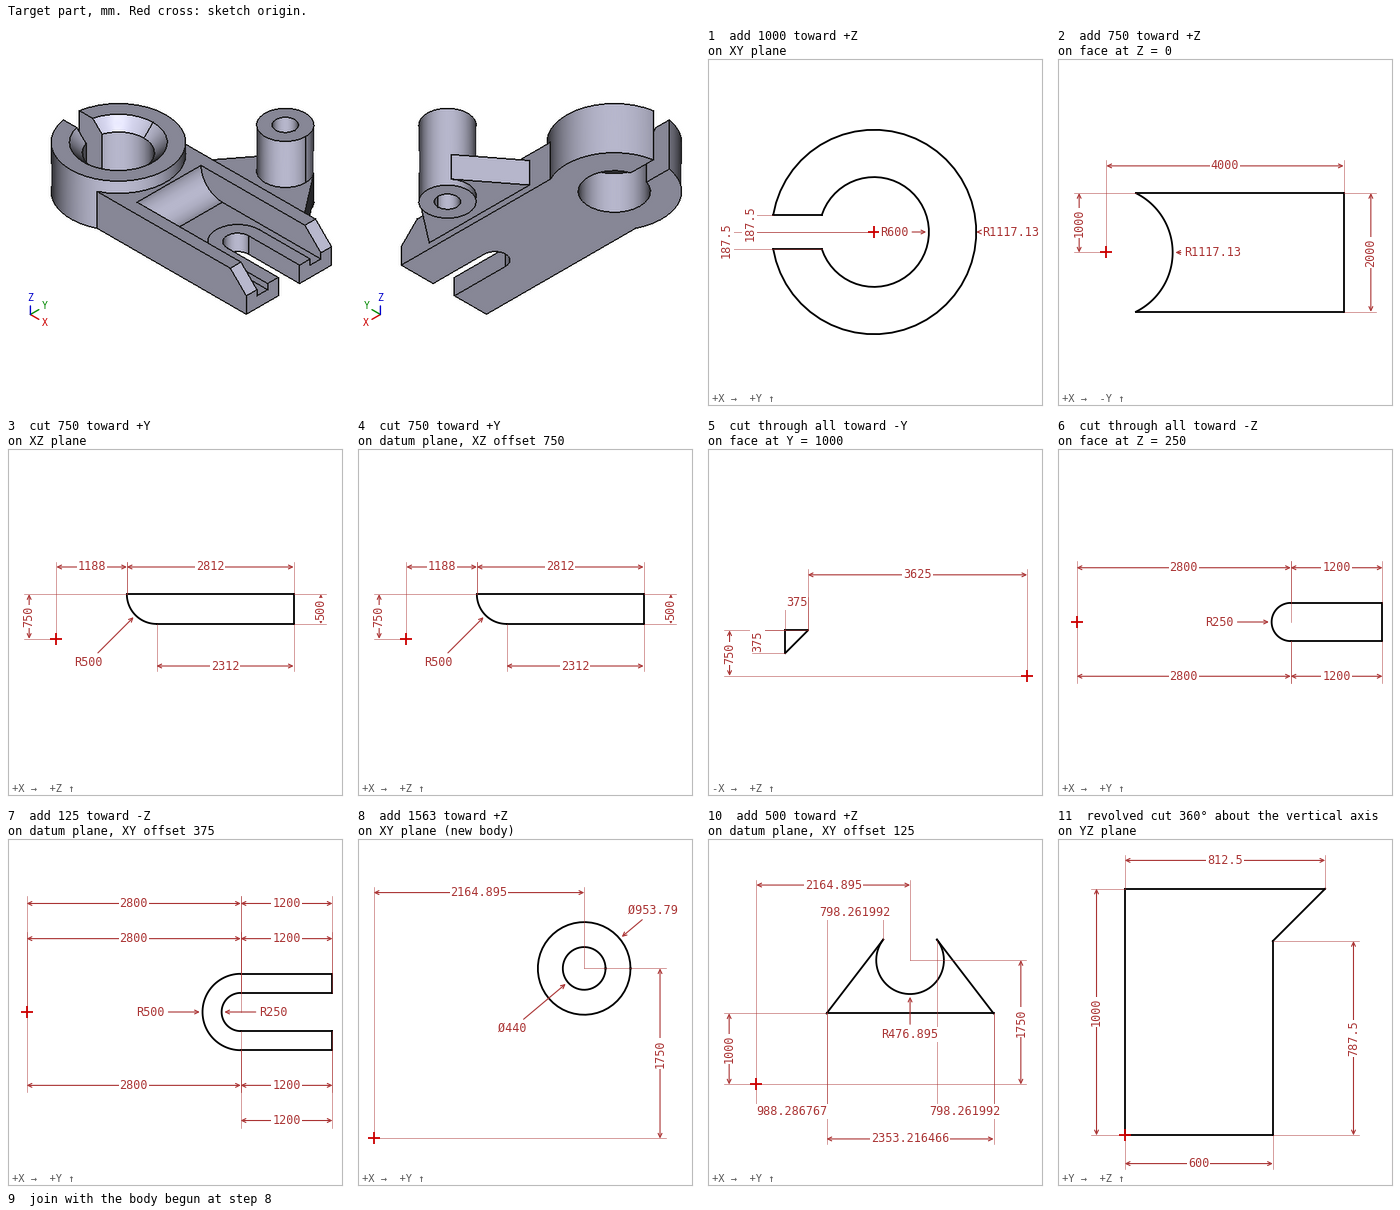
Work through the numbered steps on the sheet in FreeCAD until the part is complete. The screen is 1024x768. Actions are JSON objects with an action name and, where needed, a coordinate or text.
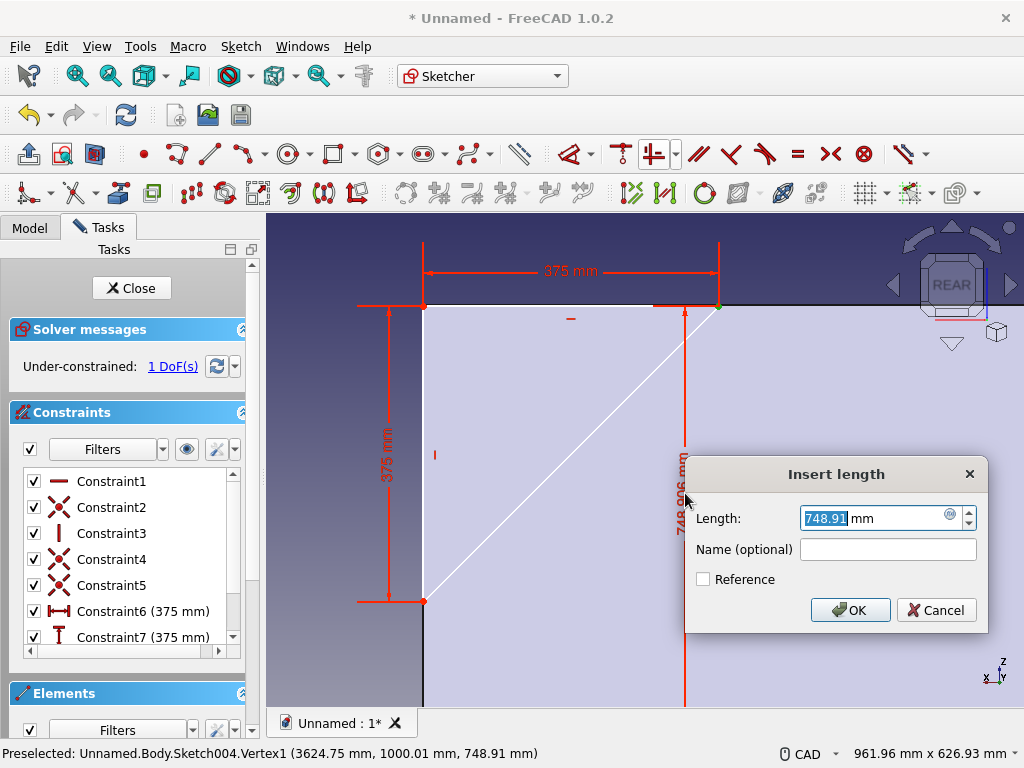
{"action": "type", "text": "750"}
{"action": "key", "text": "Return"}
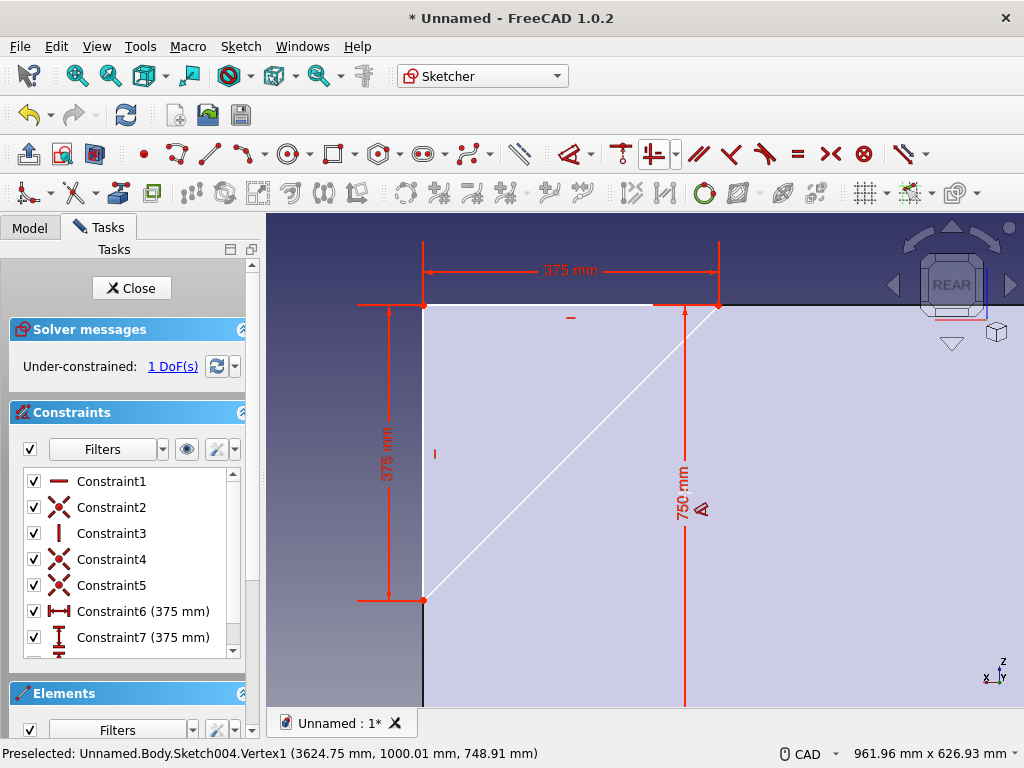
{"action": "left_click", "coordinate": [719, 305]}
{"action": "left_click", "coordinate": [789, 271]}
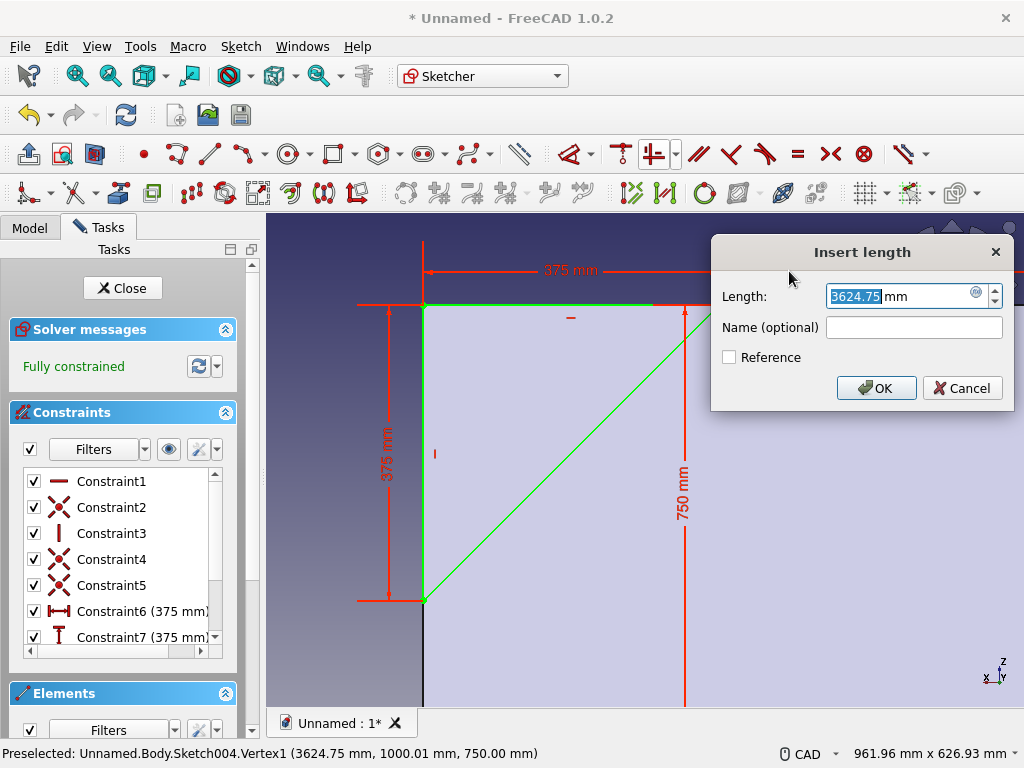
{"action": "type", "text": "3625"}
{"action": "key", "text": "Return"}
{"action": "key", "text": "Escape"}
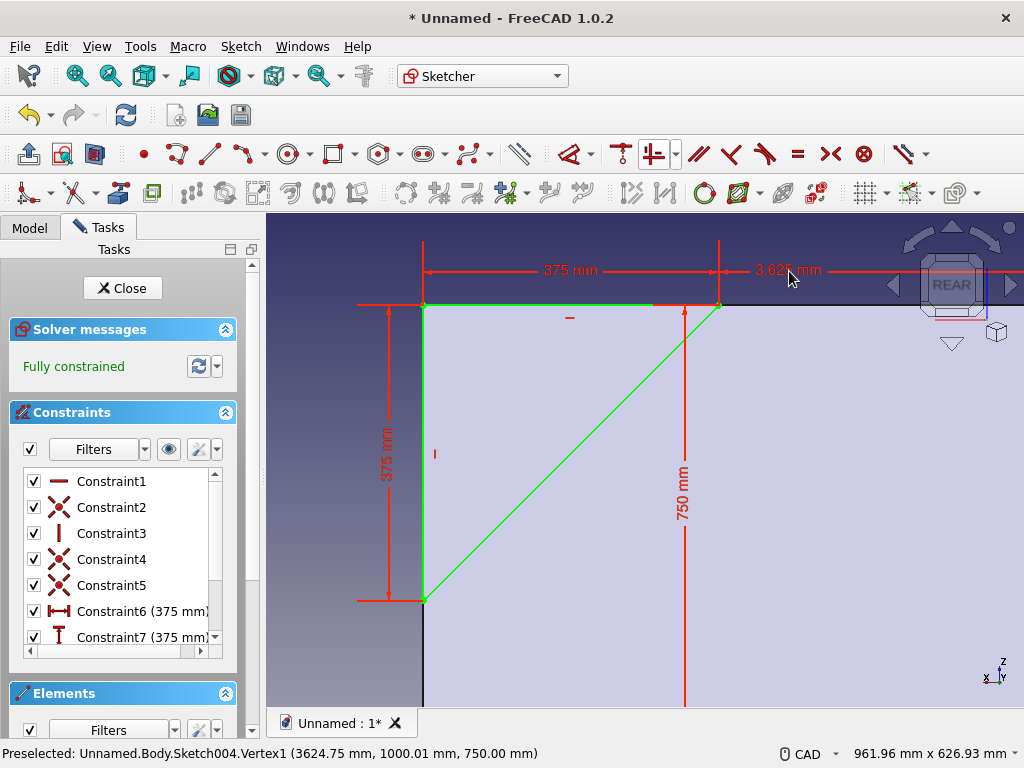
{"action": "left_click", "coordinate": [123, 288]}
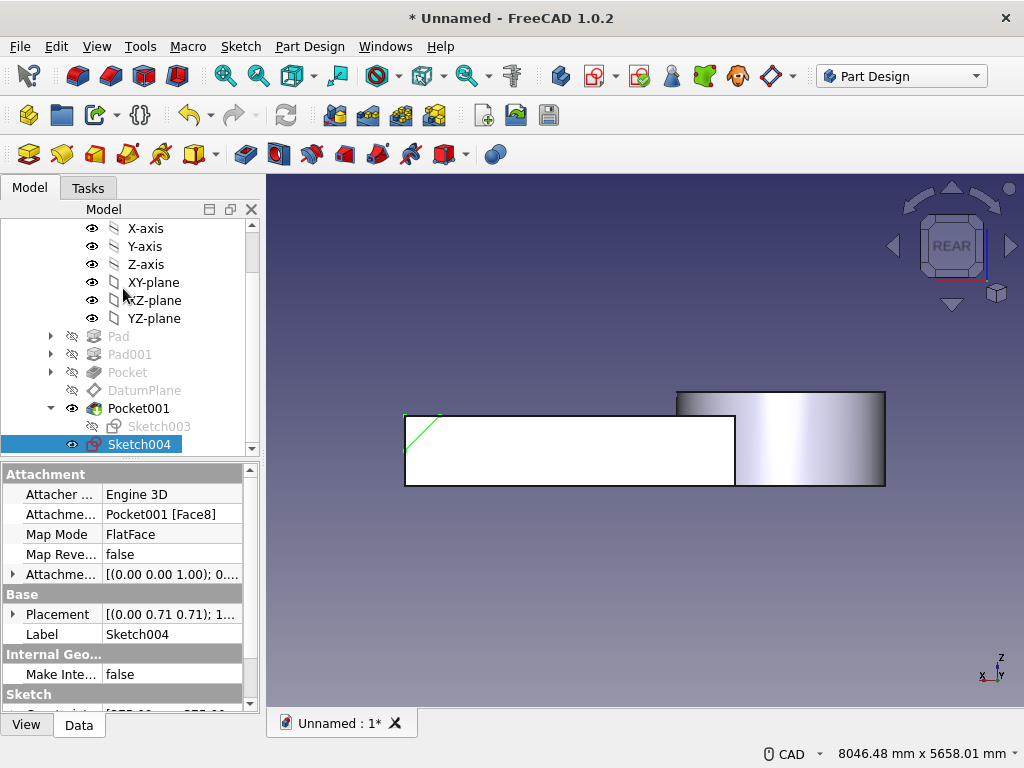
{"action": "left_click", "coordinate": [246, 154]}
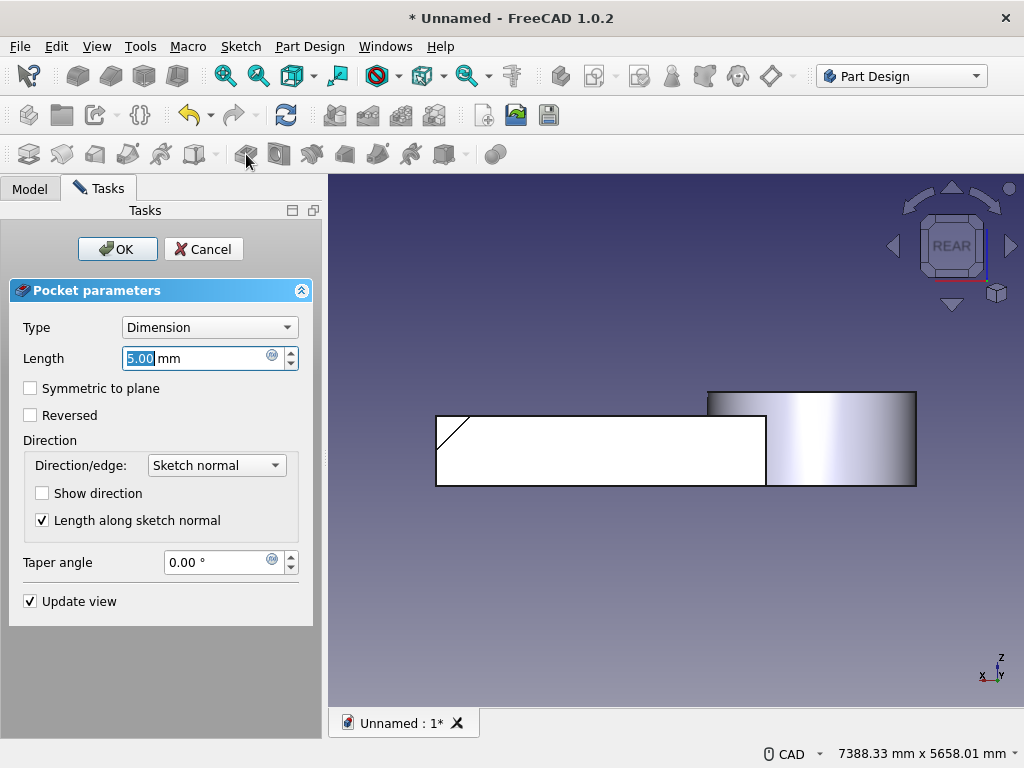
{"action": "left_click", "coordinate": [210, 328]}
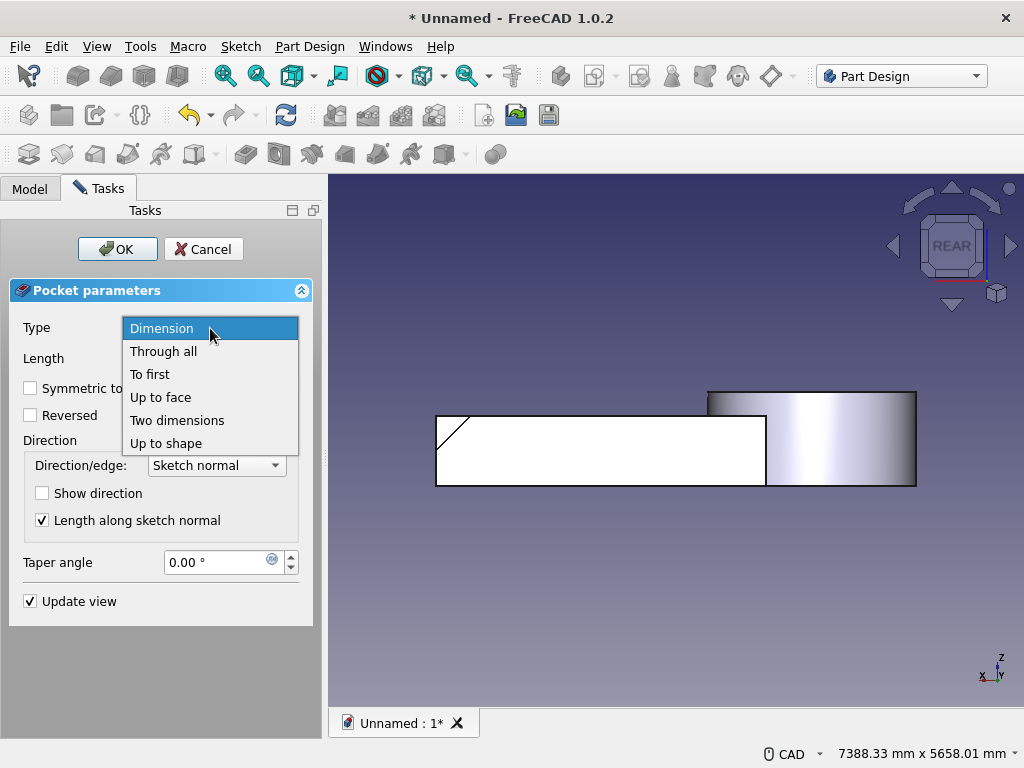
{"action": "left_click", "coordinate": [208, 352]}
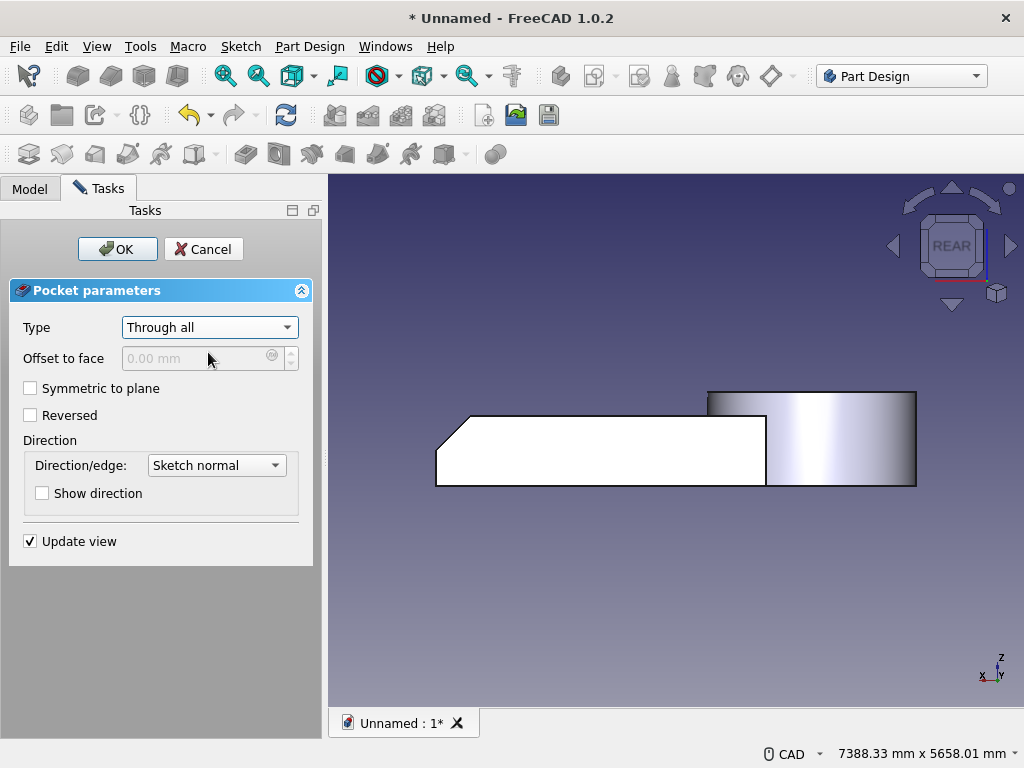
{"action": "left_click", "coordinate": [118, 249]}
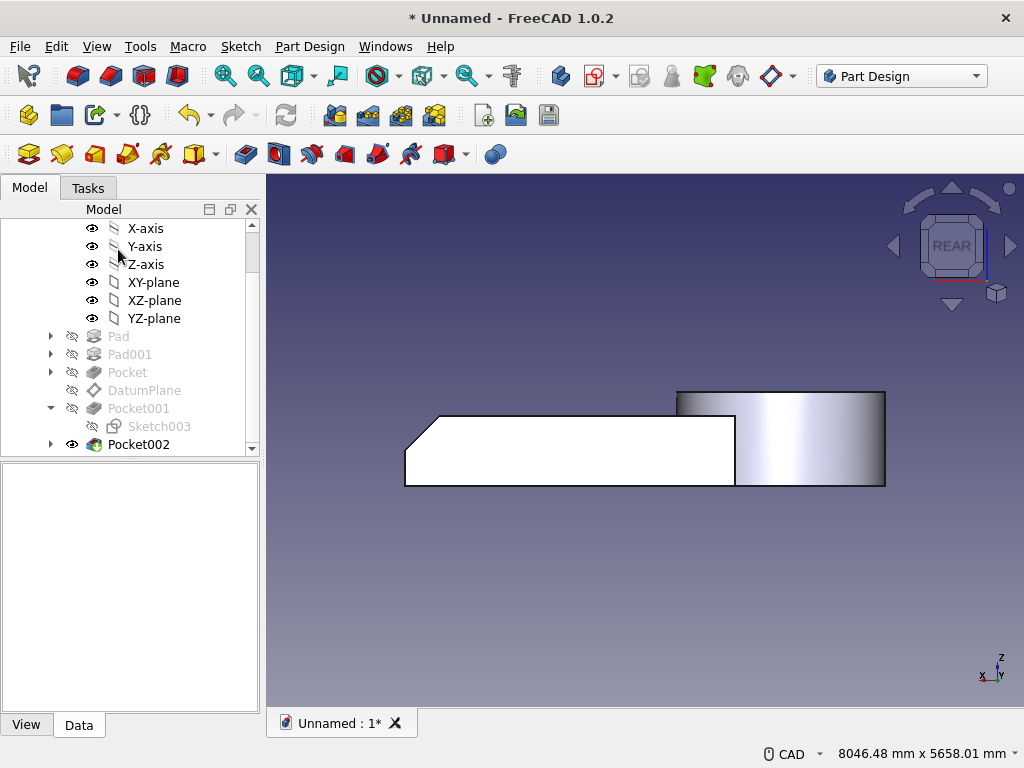
{"action": "key", "text": "0"}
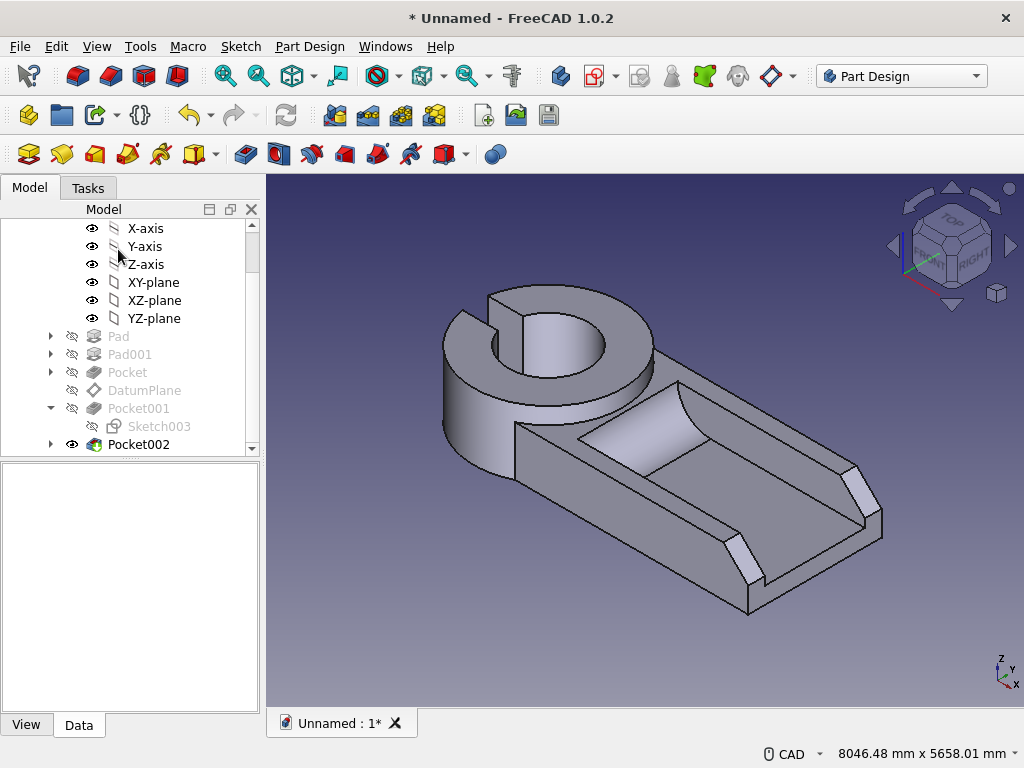
{"action": "left_click", "coordinate": [760, 524]}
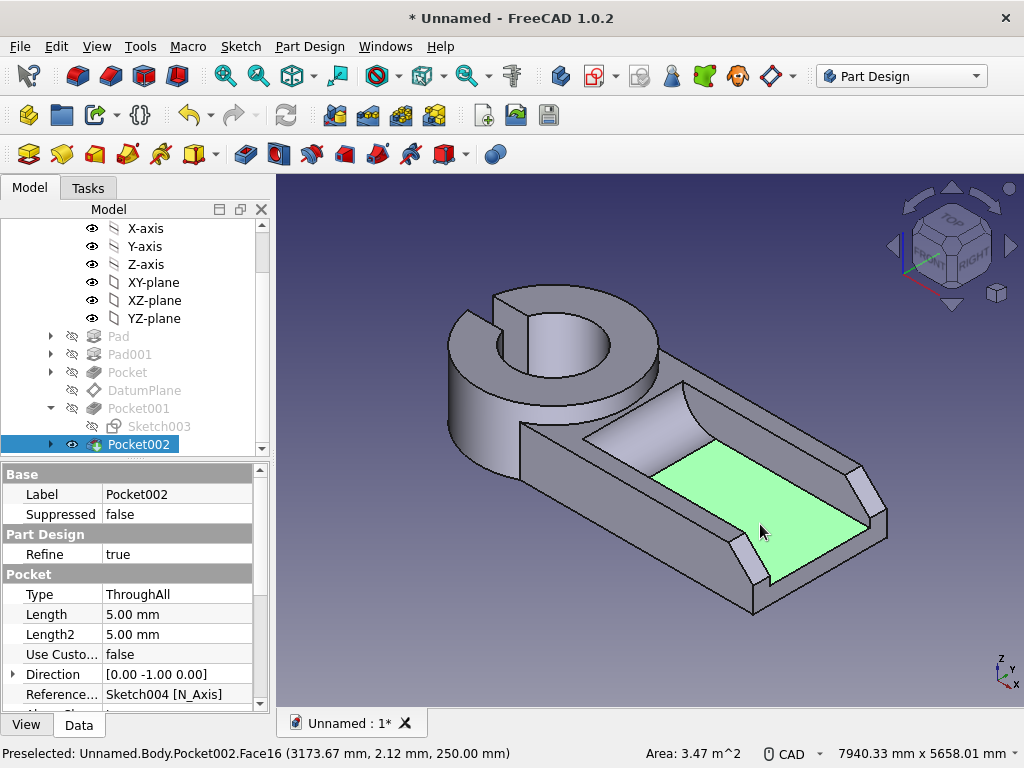
{"action": "left_click", "coordinate": [594, 76]}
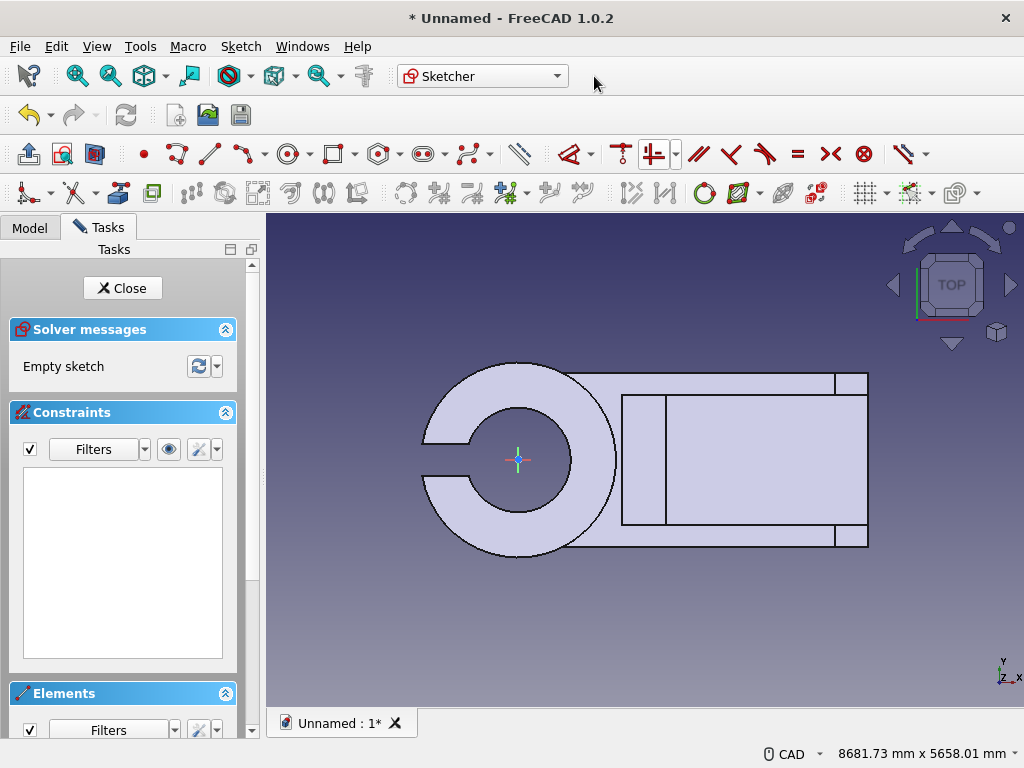
{"action": "scroll", "coordinate": [576, 460], "scroll_direction": "down", "scroll_amount": 5}